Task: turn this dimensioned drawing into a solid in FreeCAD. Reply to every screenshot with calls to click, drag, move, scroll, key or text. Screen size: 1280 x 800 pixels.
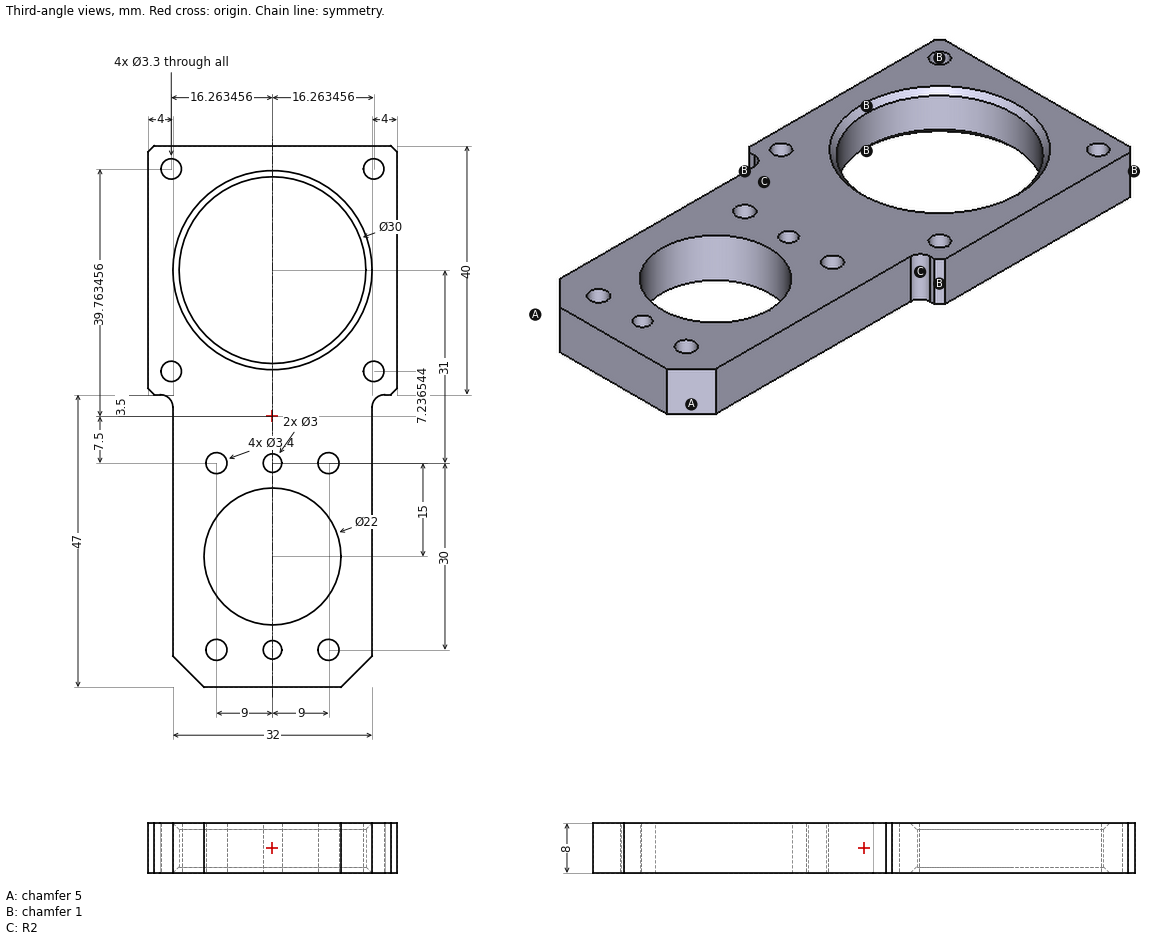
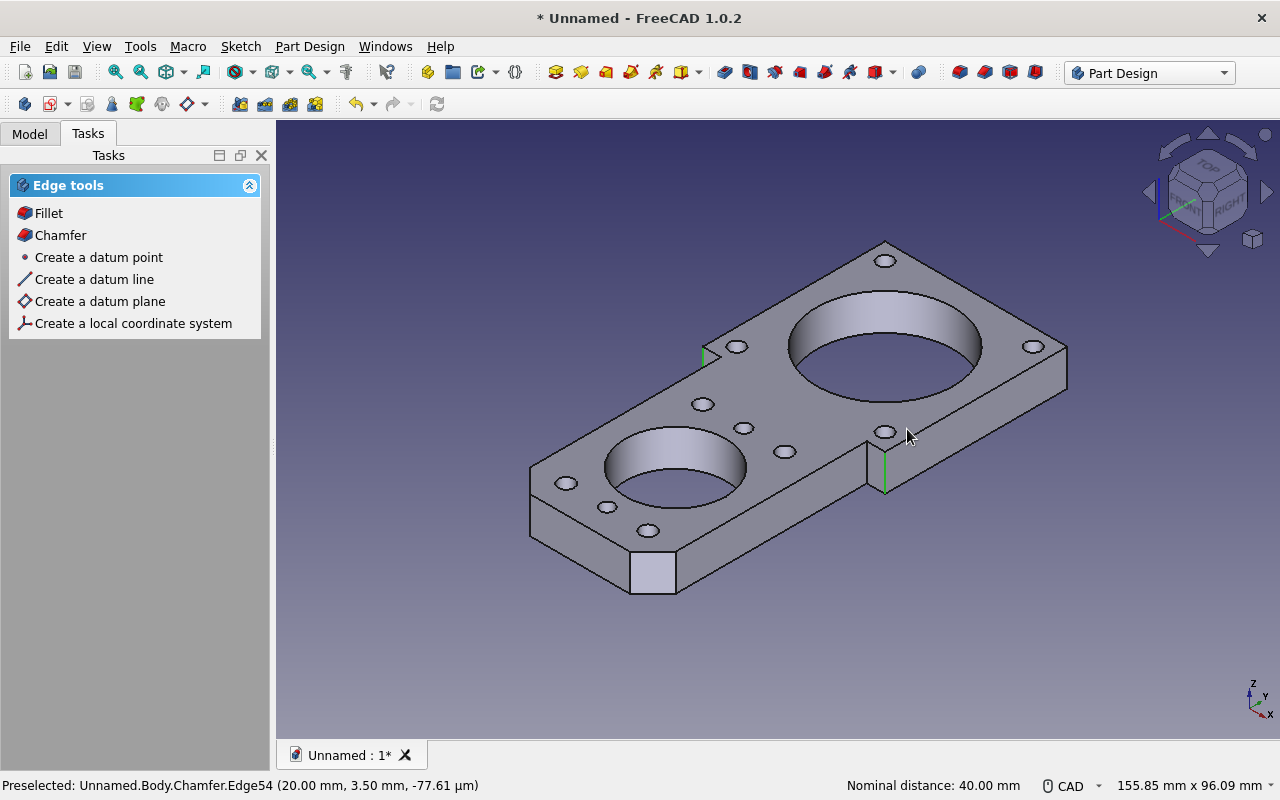
click(817, 306, ctrl)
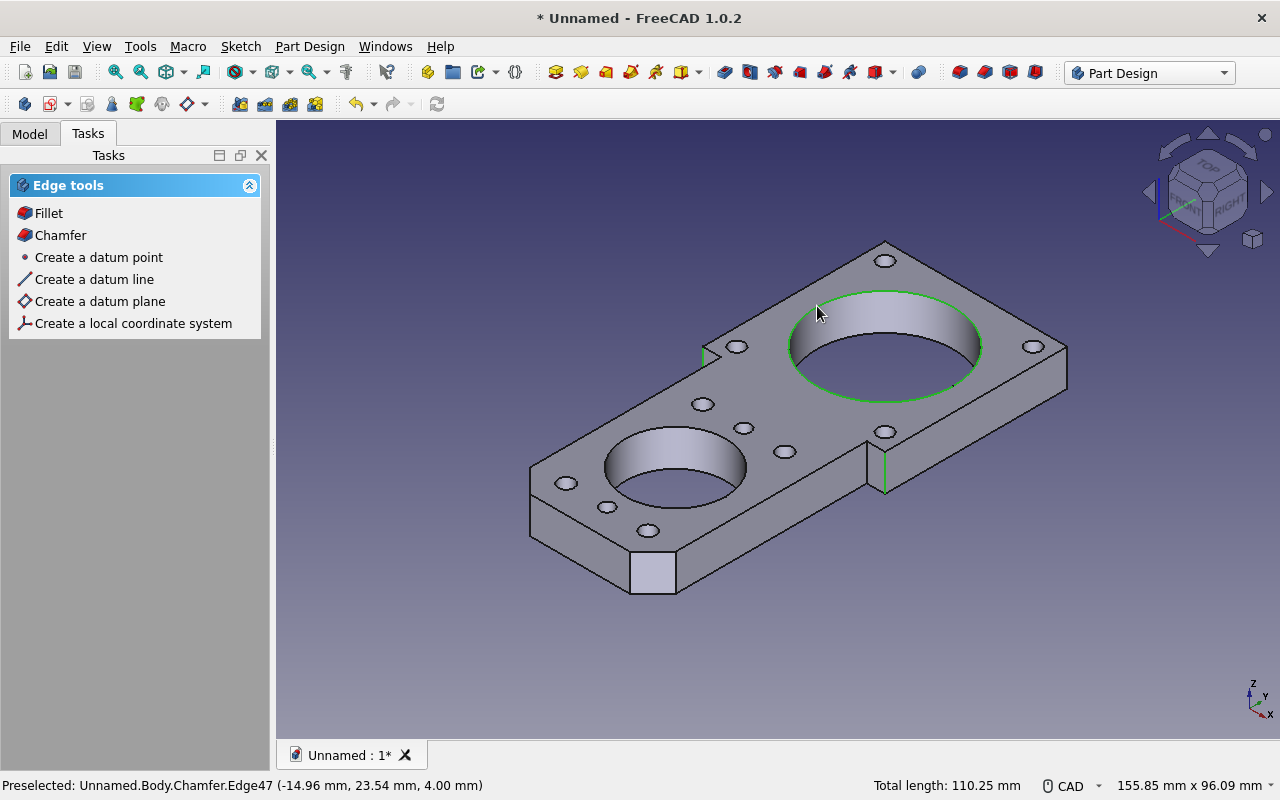
key(2)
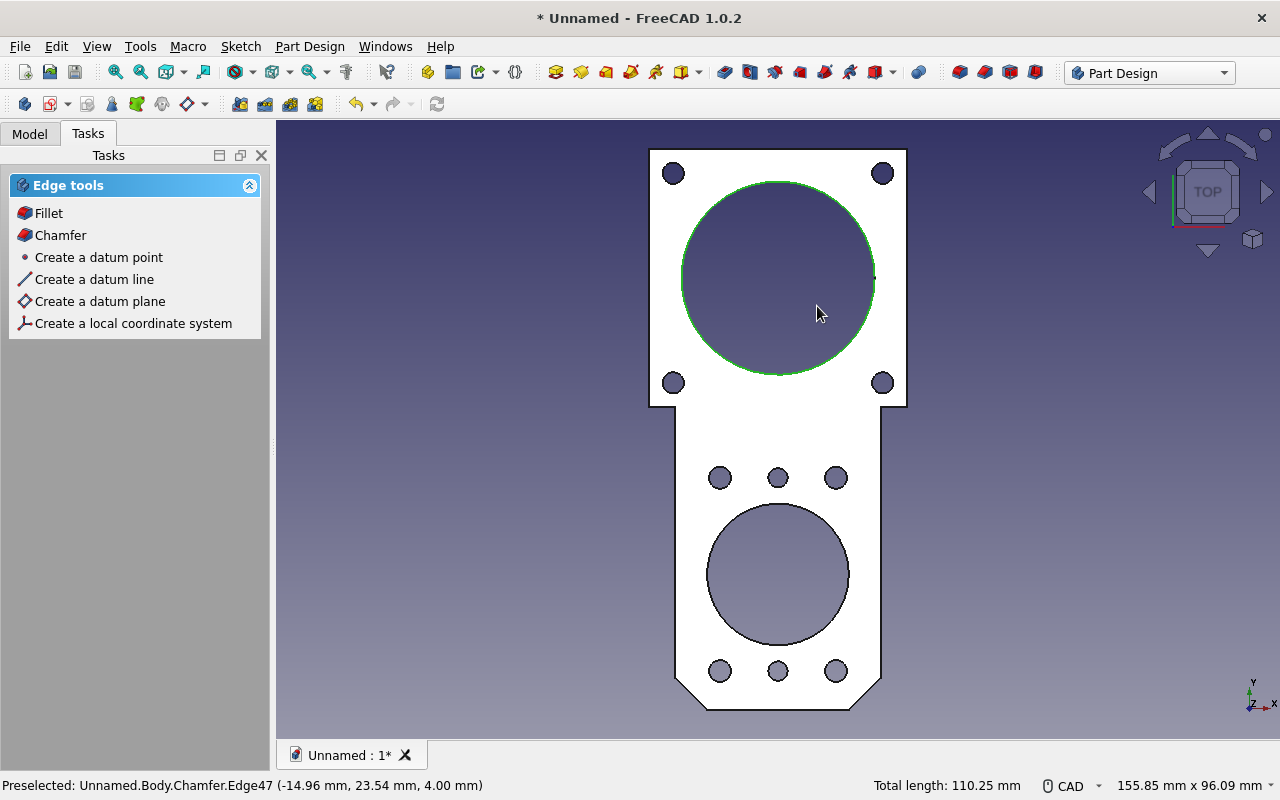
key(1)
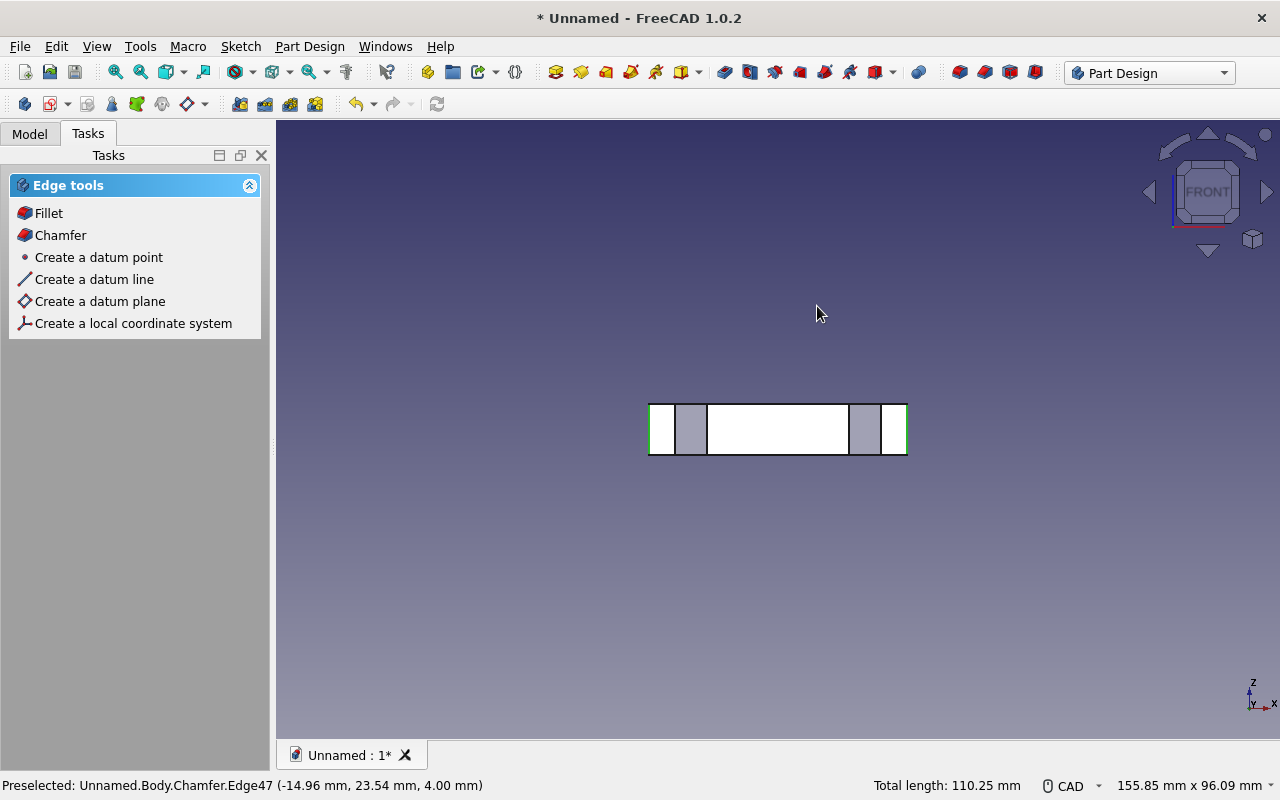
key(v)
key(f)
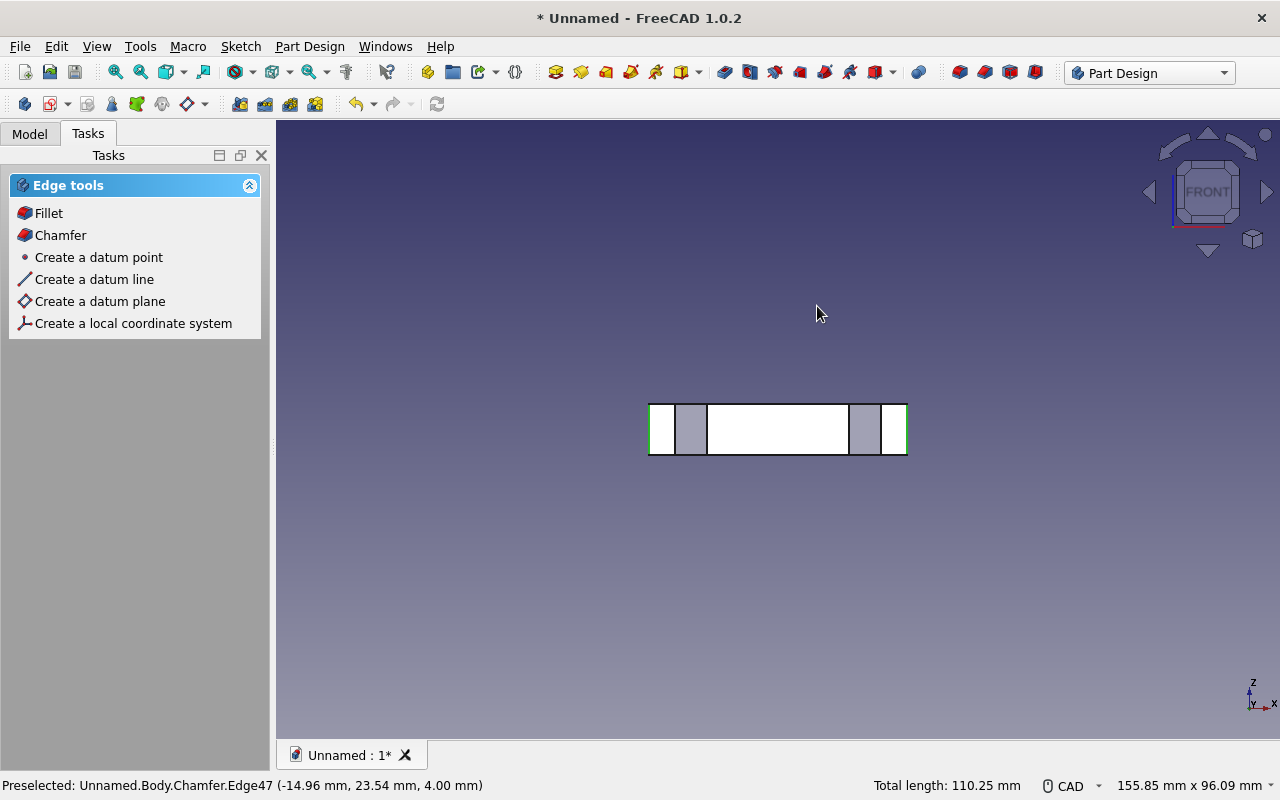
key(3)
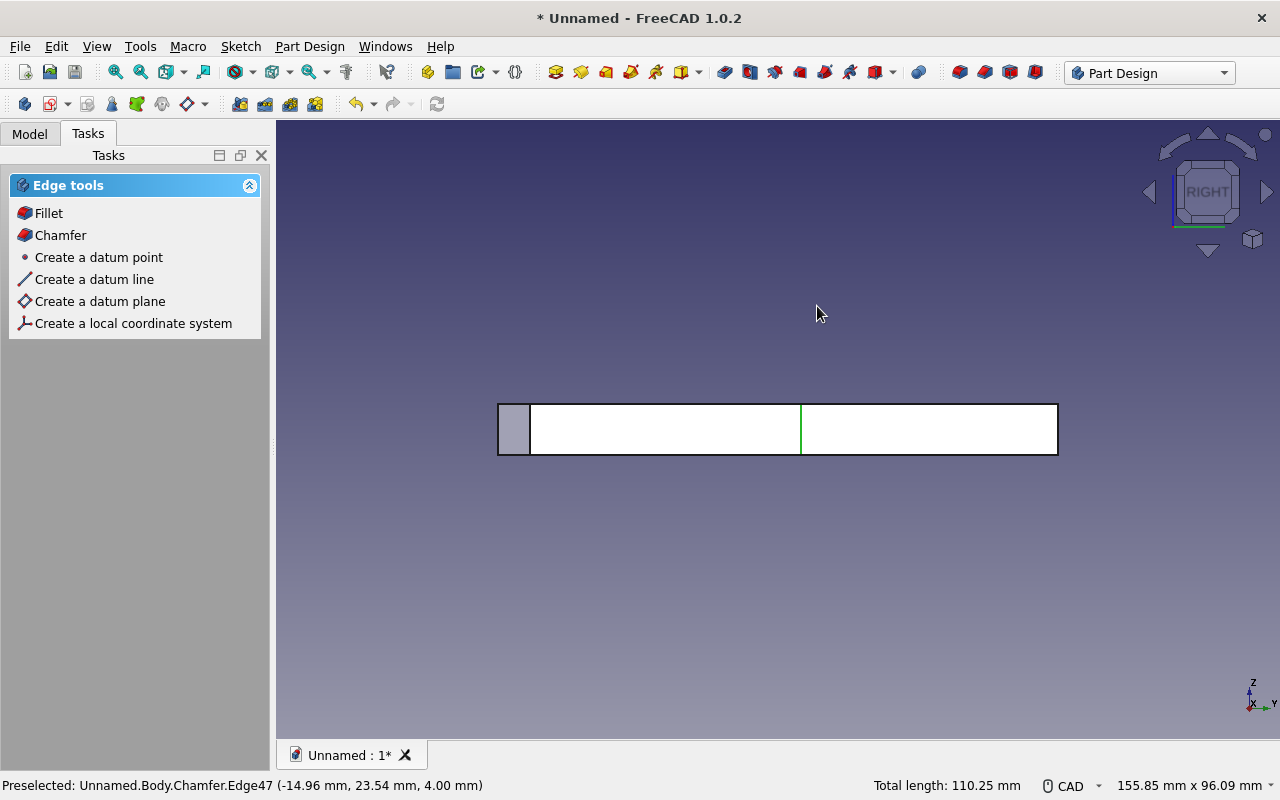
click(1058, 428, ctrl)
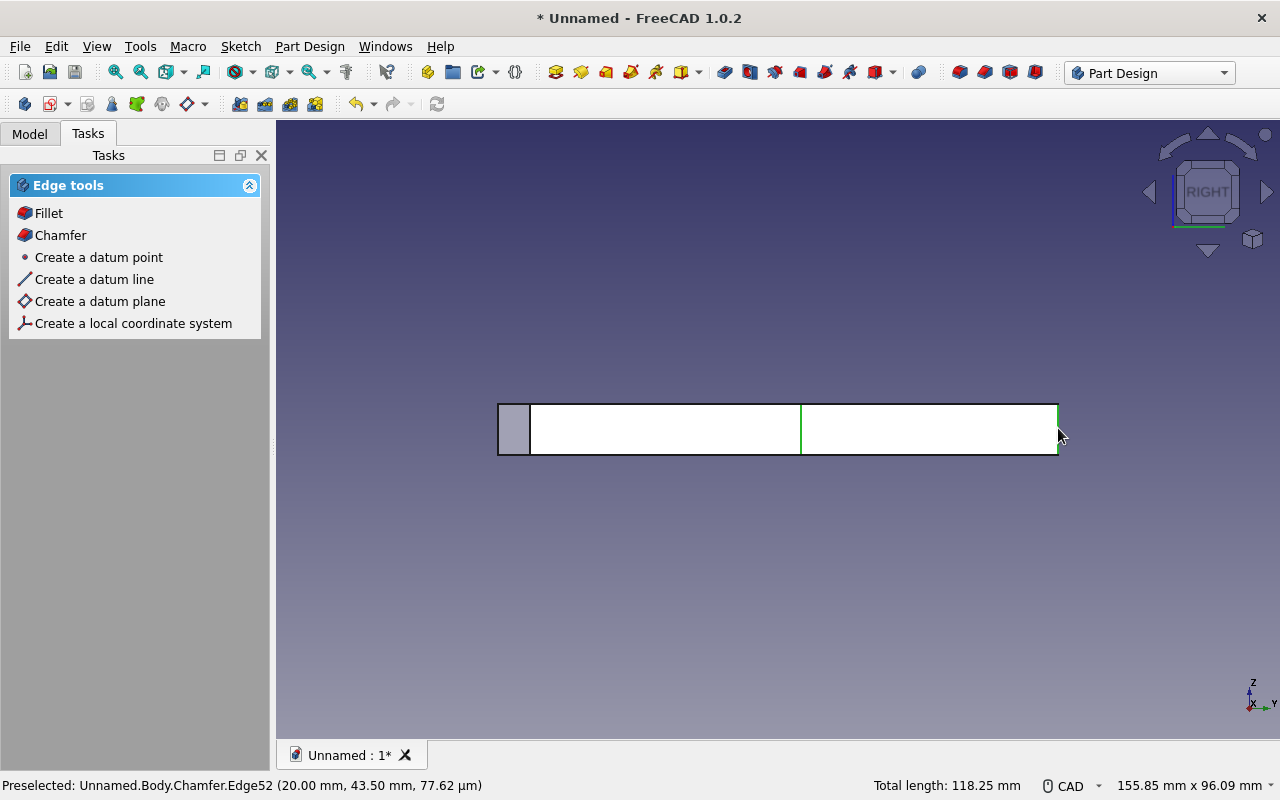
key(5)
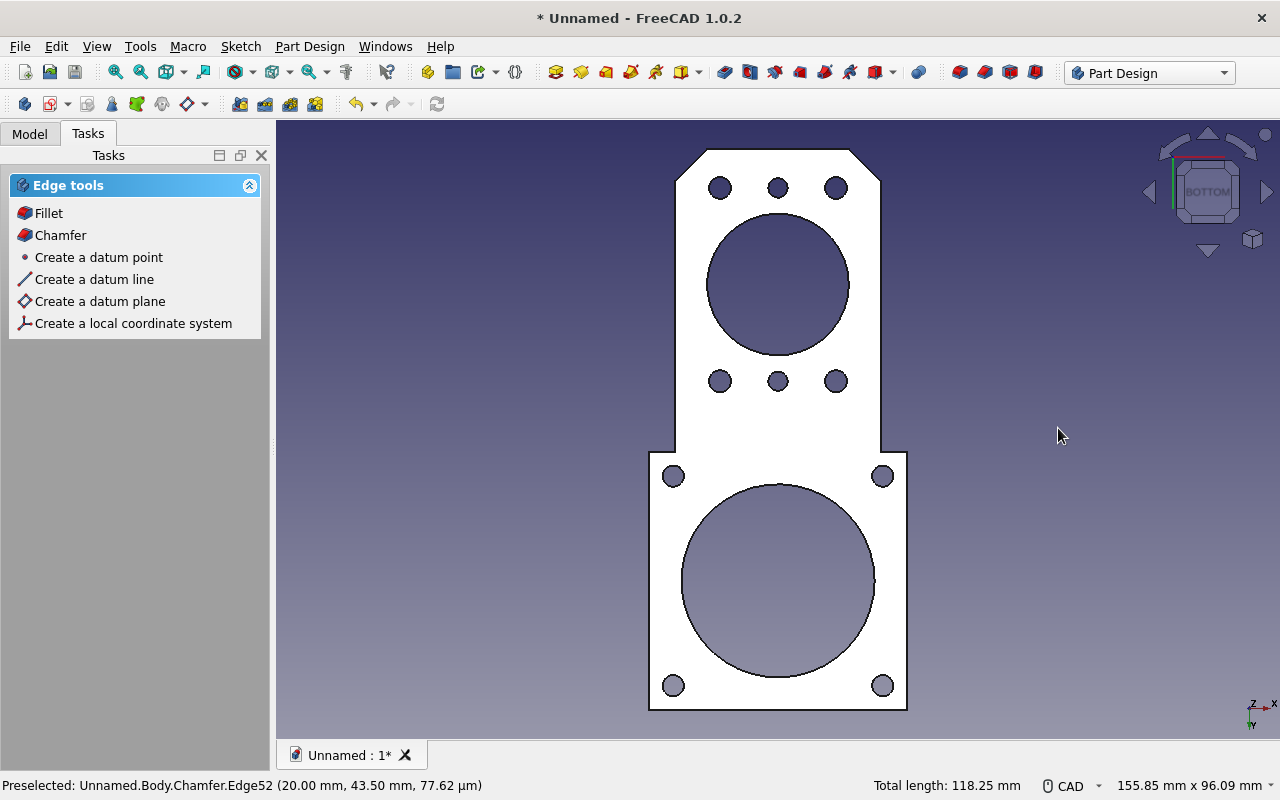
click(681, 580, ctrl)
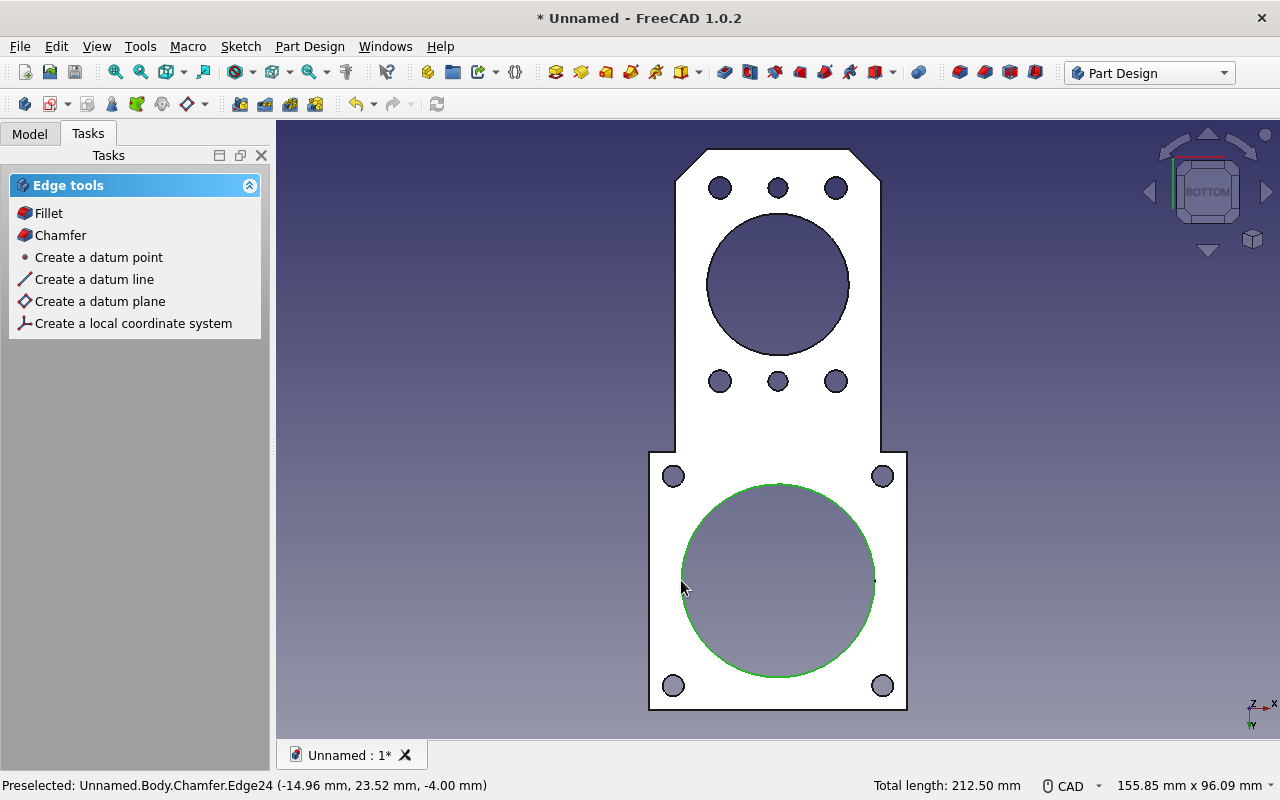
key(4)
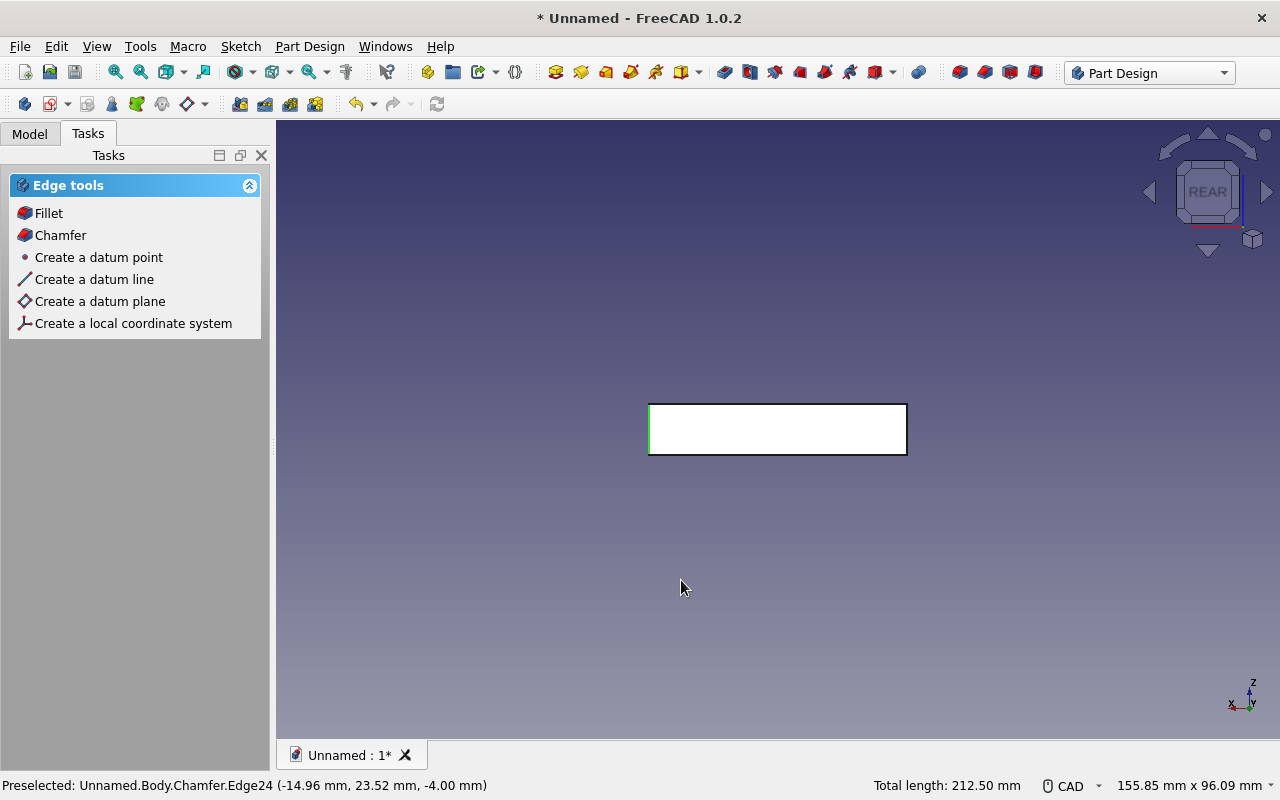
key(v)
key(f)